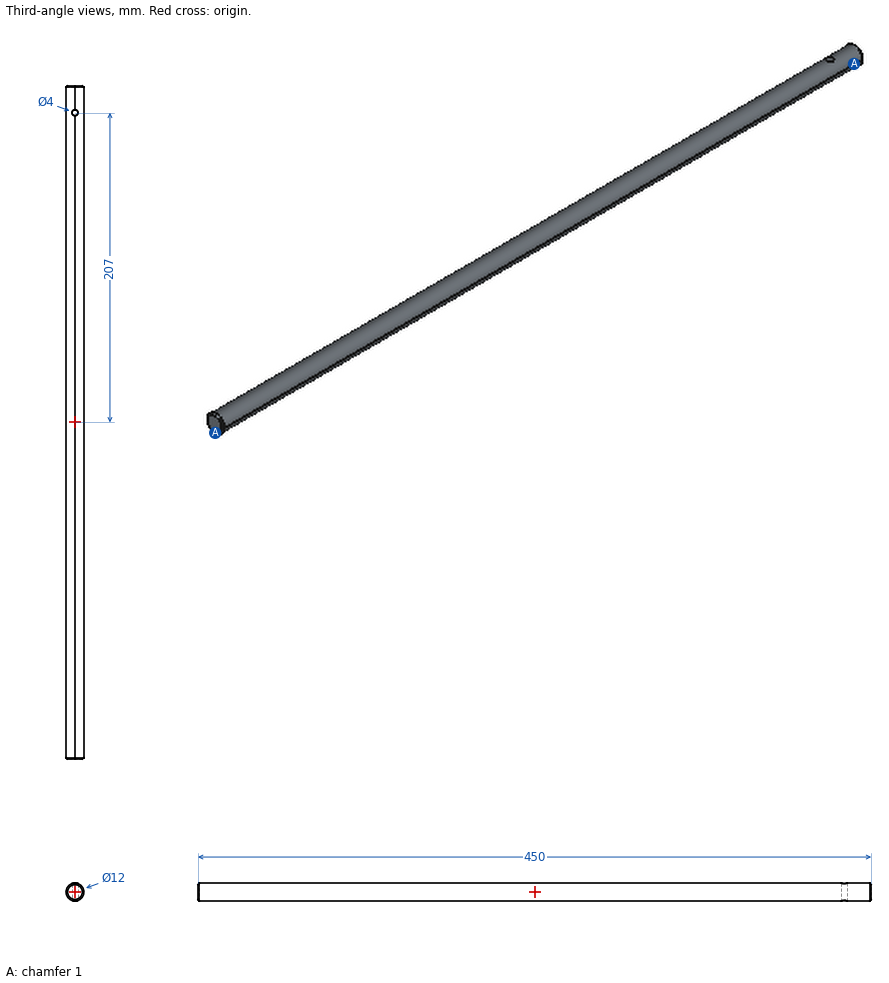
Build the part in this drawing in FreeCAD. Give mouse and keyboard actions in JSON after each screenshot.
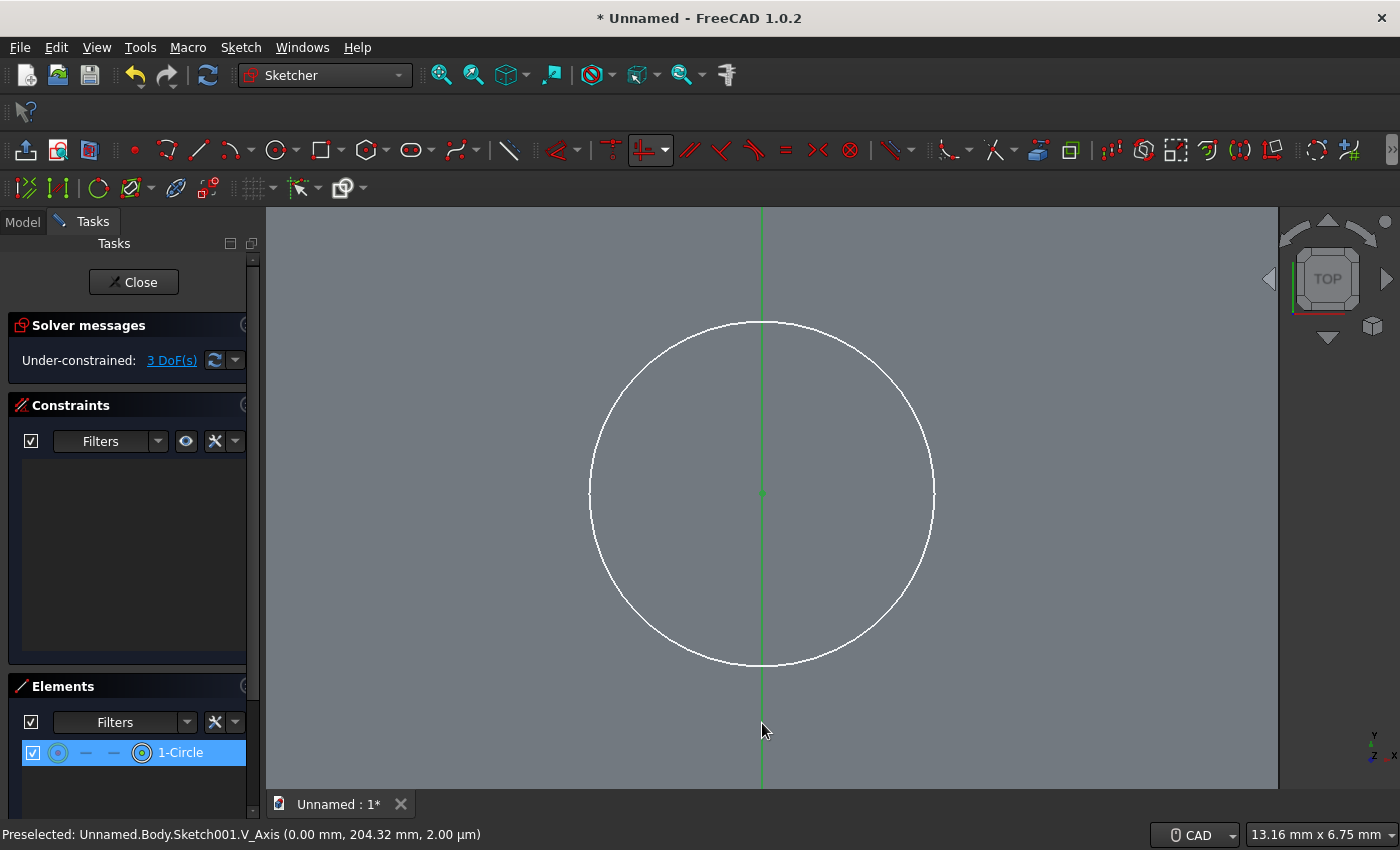
{"action": "key", "text": "c"}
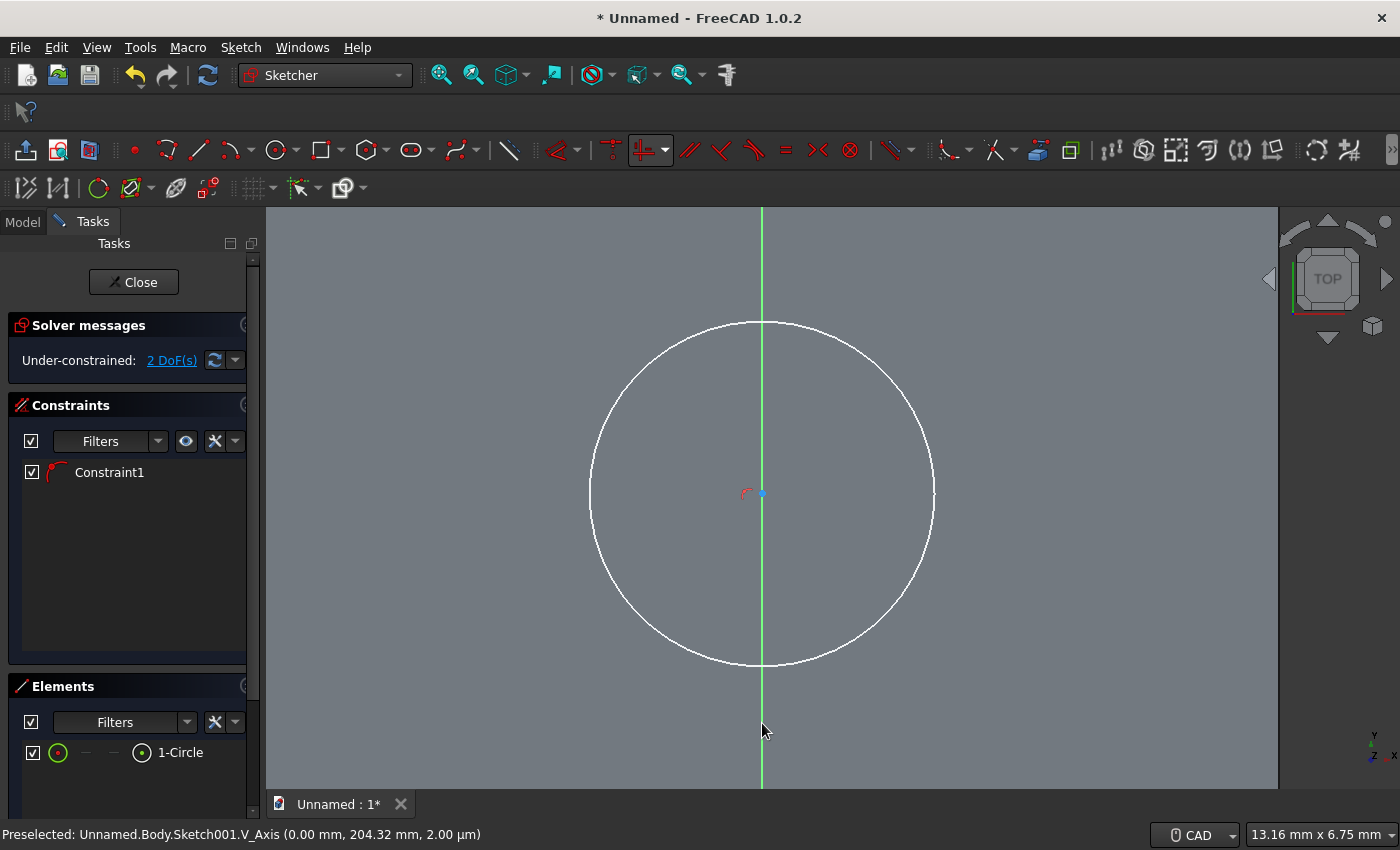
{"action": "key", "text": "d"}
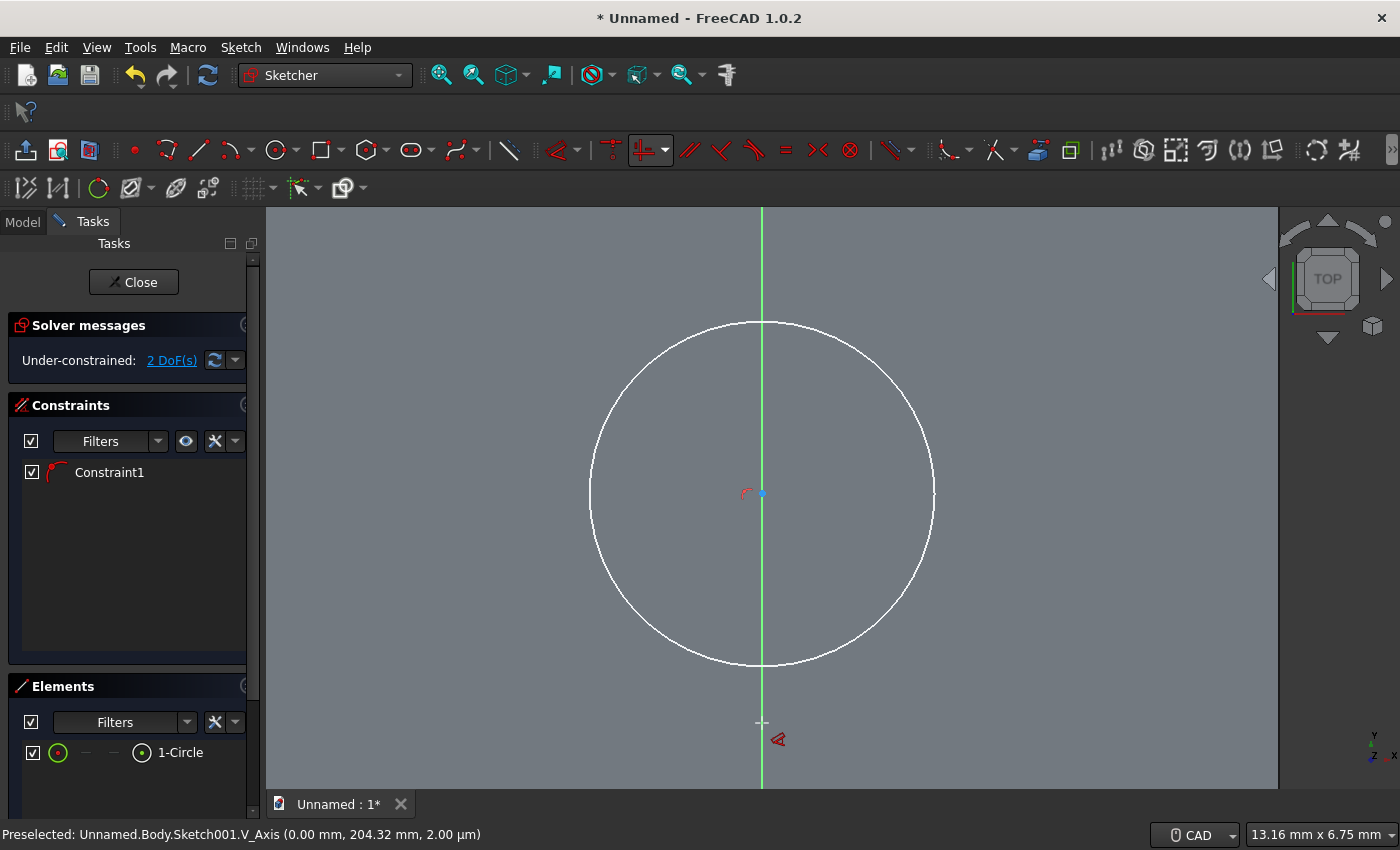
{"action": "left_click", "coordinate": [884, 372]}
{"action": "left_click", "coordinate": [907, 349]}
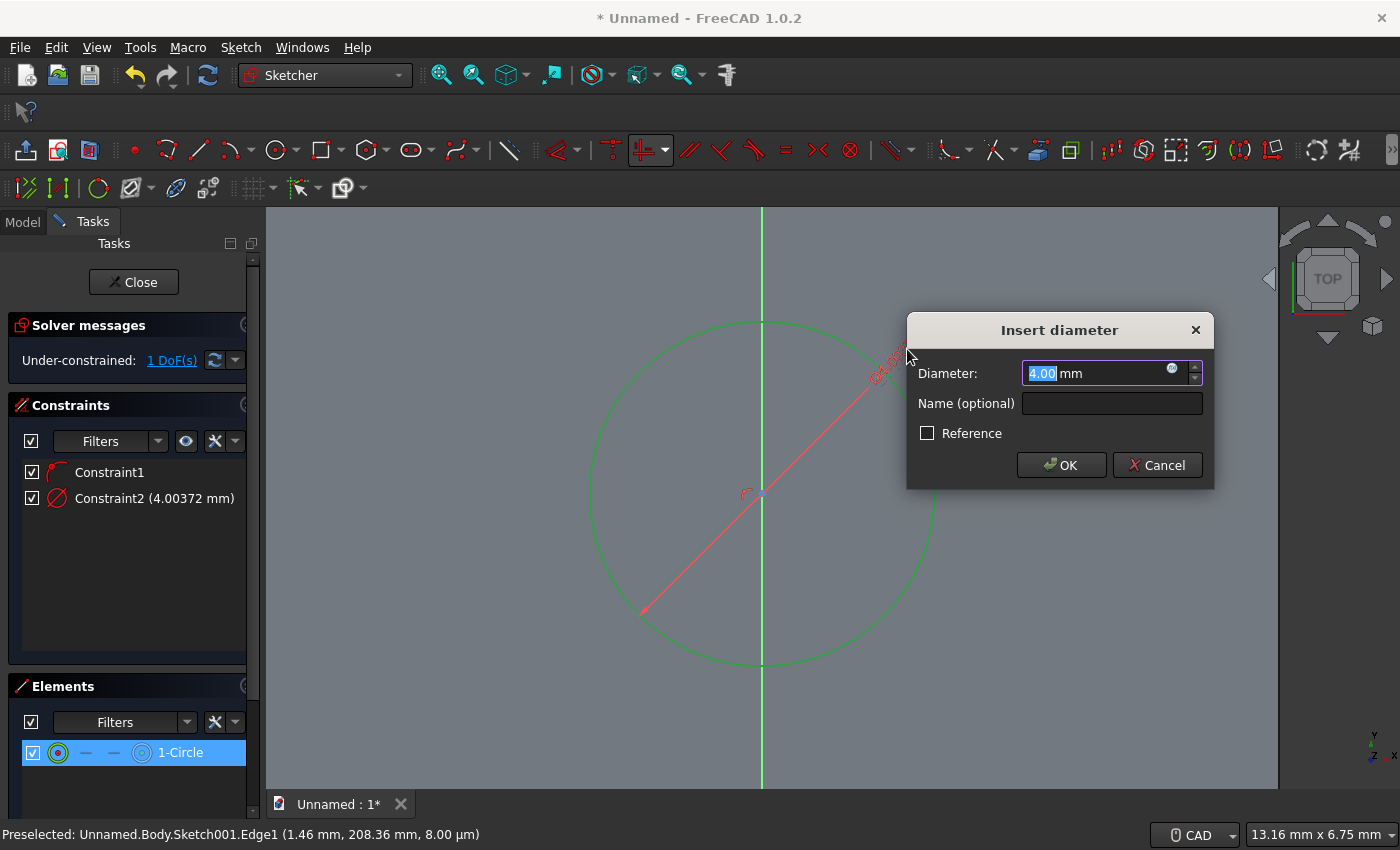
{"action": "type", "text": "4"}
{"action": "key", "text": "Return"}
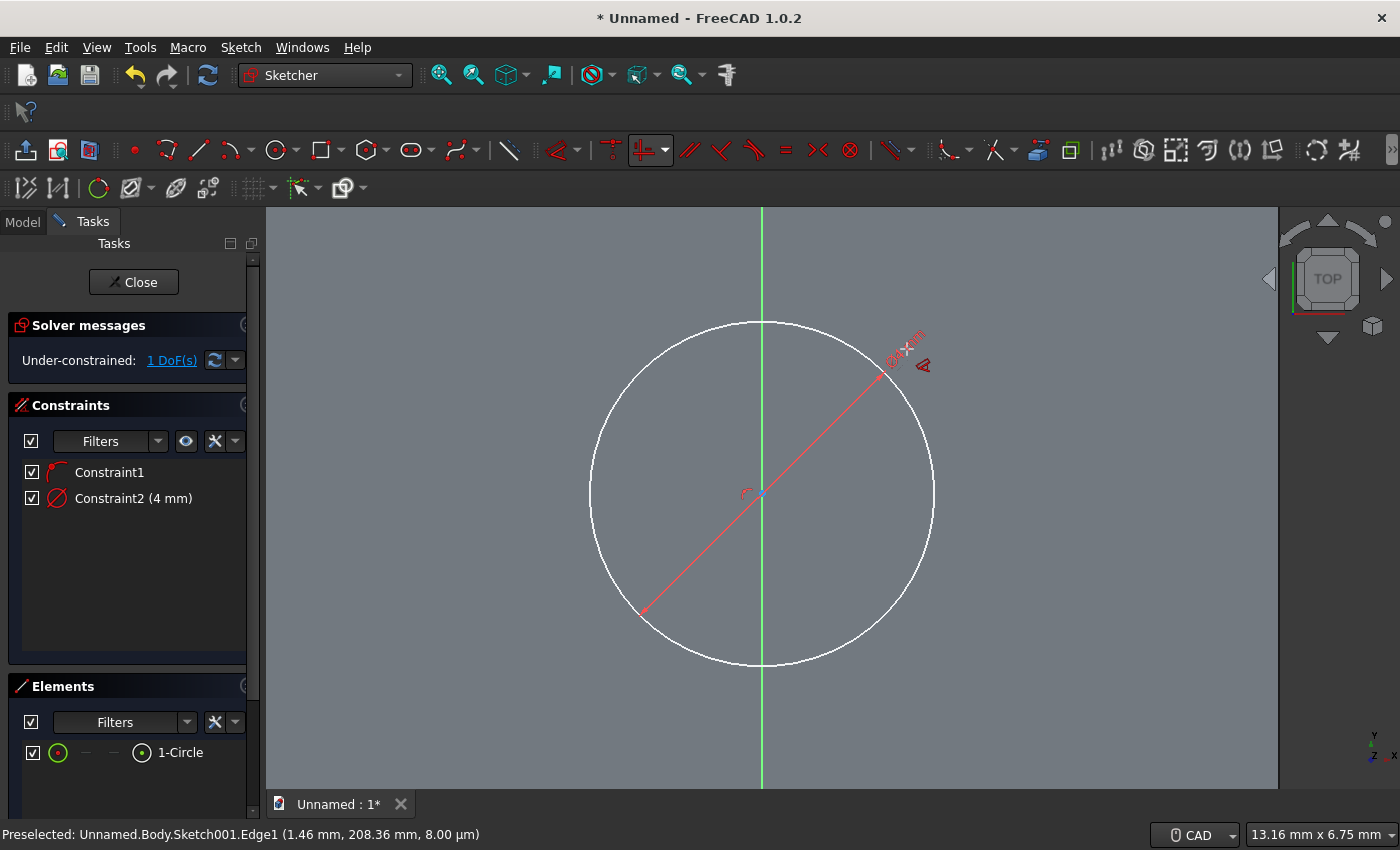
{"action": "left_click", "coordinate": [762, 494]}
{"action": "left_click", "coordinate": [796, 627]}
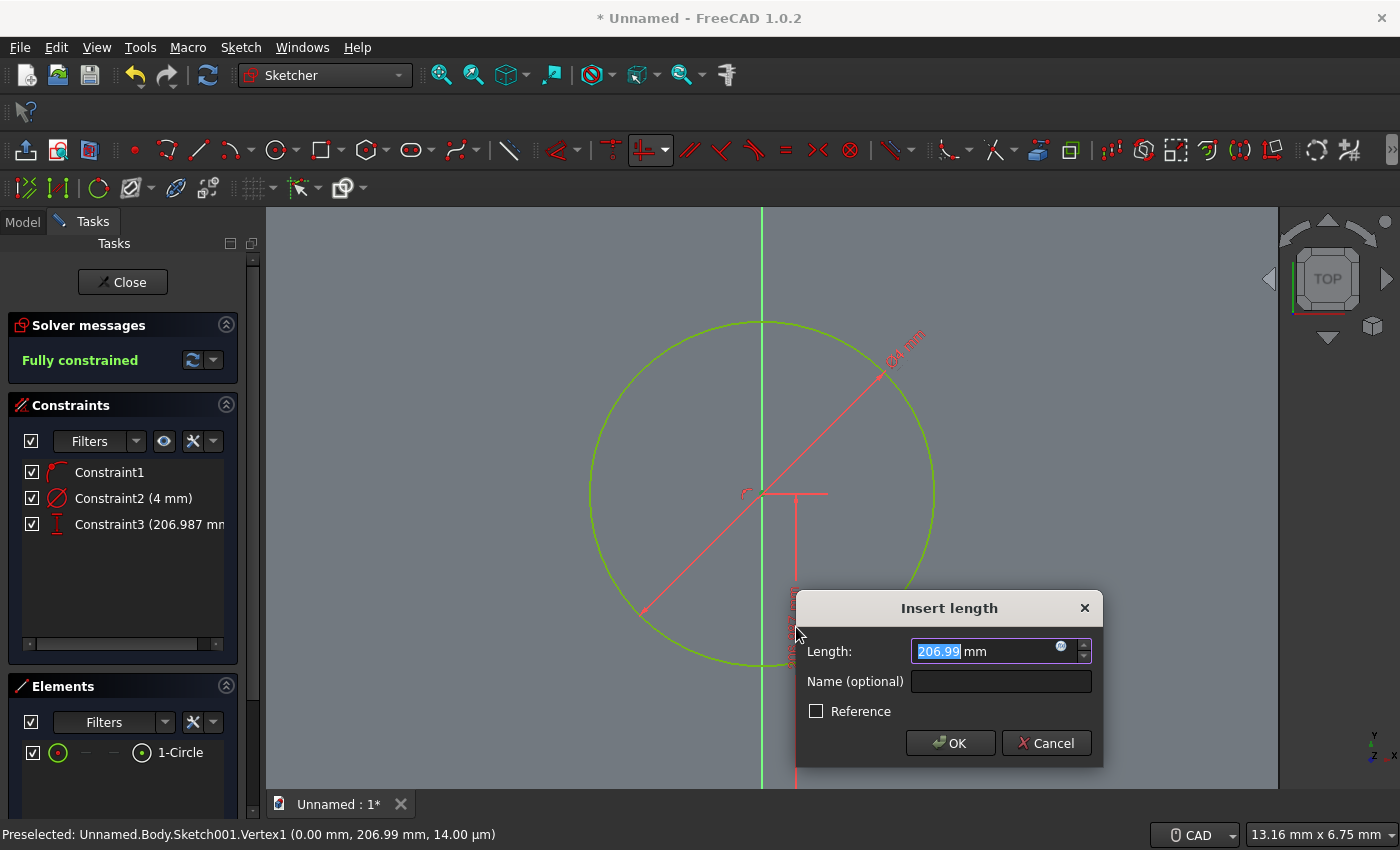
{"action": "type", "text": "207"}
{"action": "key", "text": "Return"}
{"action": "key", "text": "Escape"}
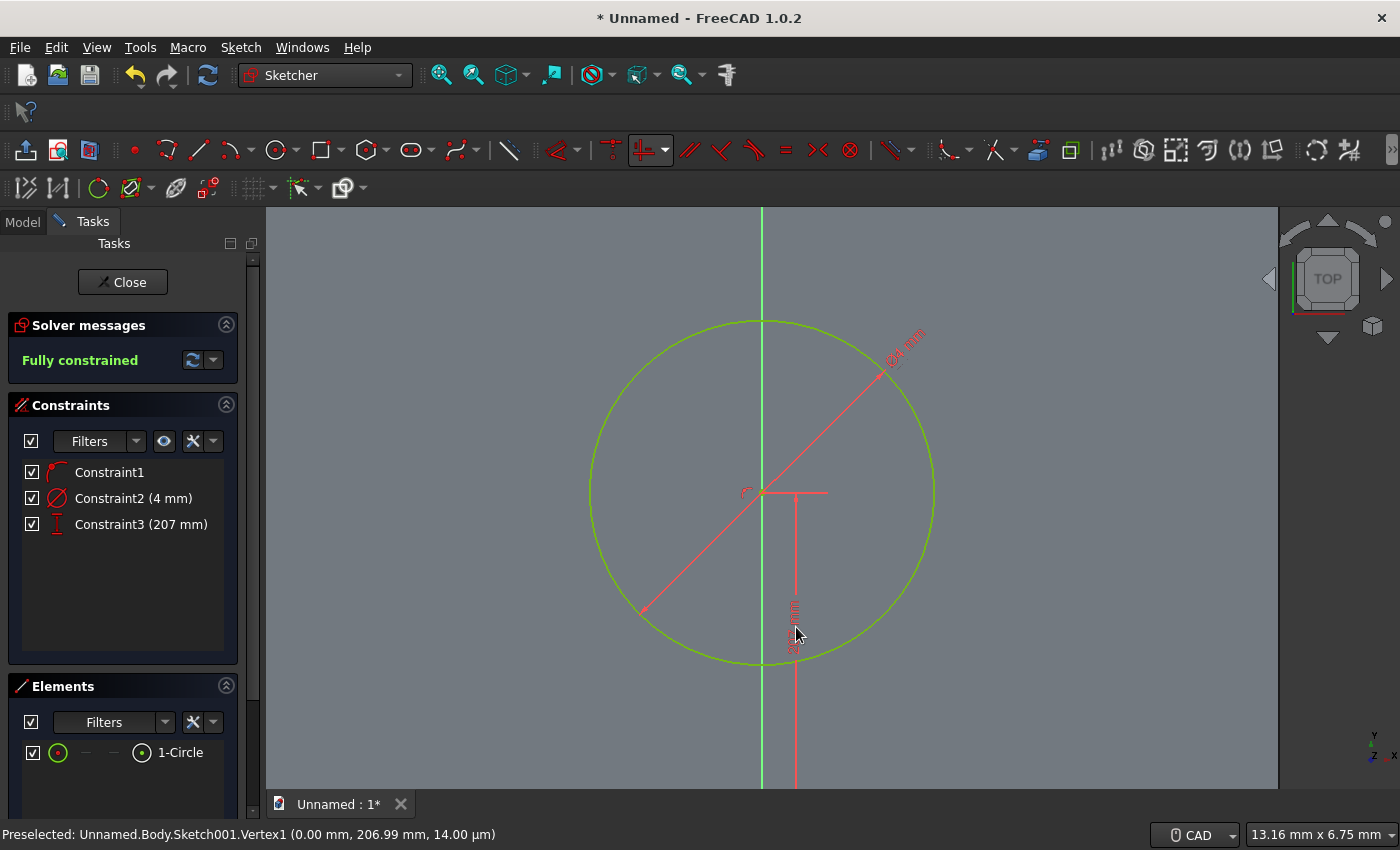
{"action": "left_click", "coordinate": [123, 282]}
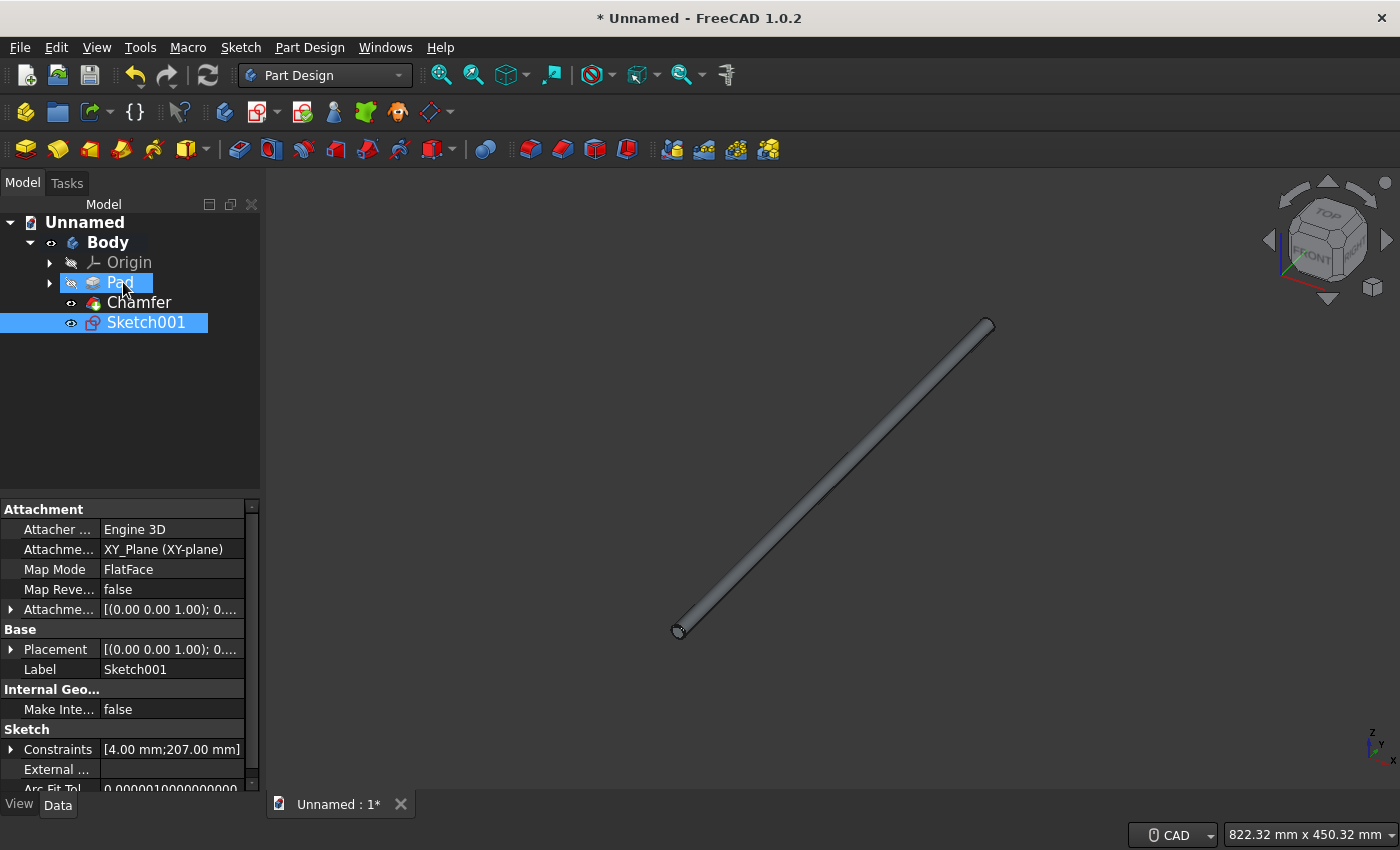
{"action": "left_click", "coordinate": [240, 150]}